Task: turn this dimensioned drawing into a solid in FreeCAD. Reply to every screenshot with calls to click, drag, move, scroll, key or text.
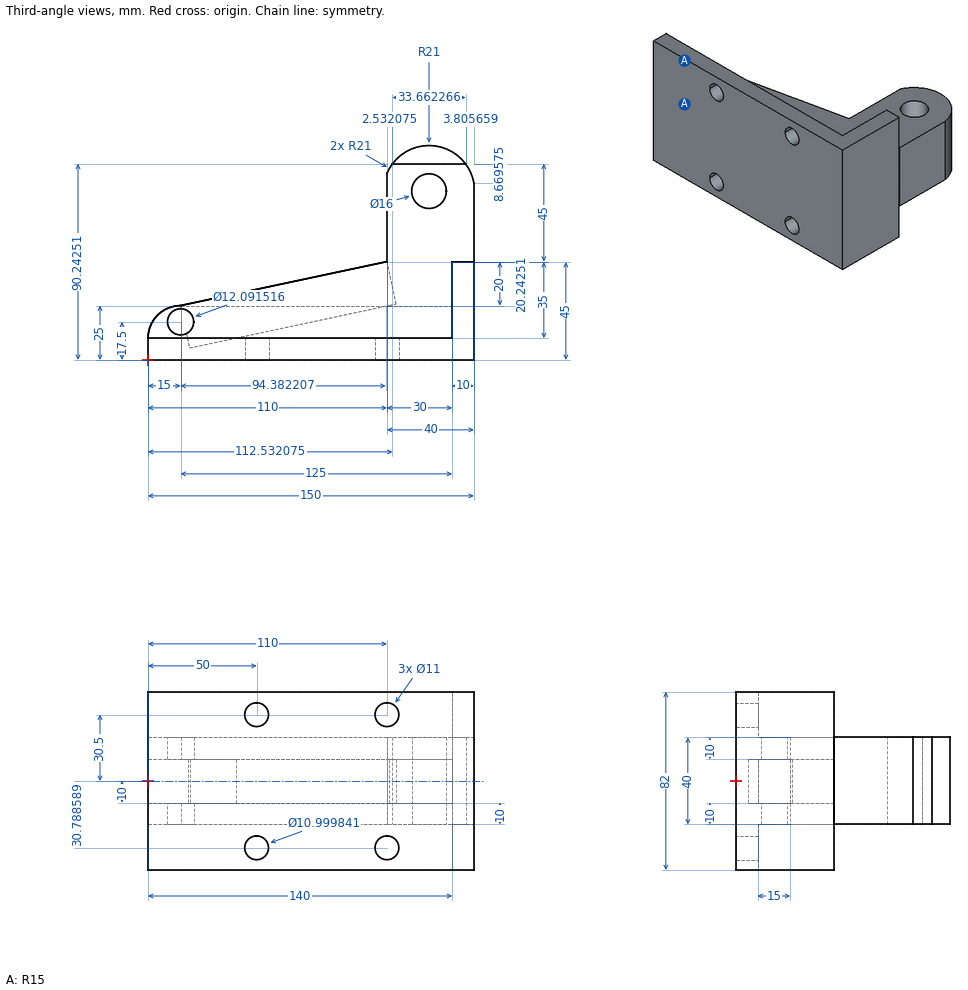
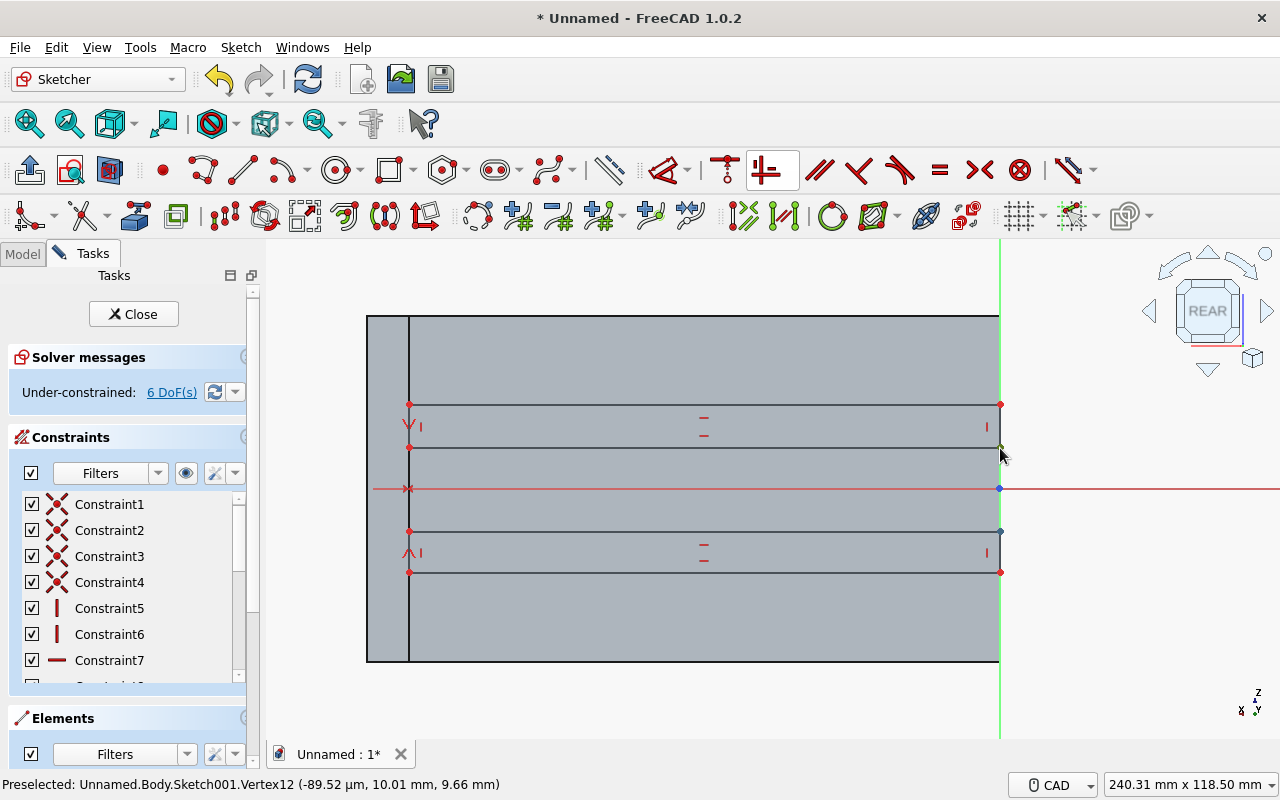
click(470, 489)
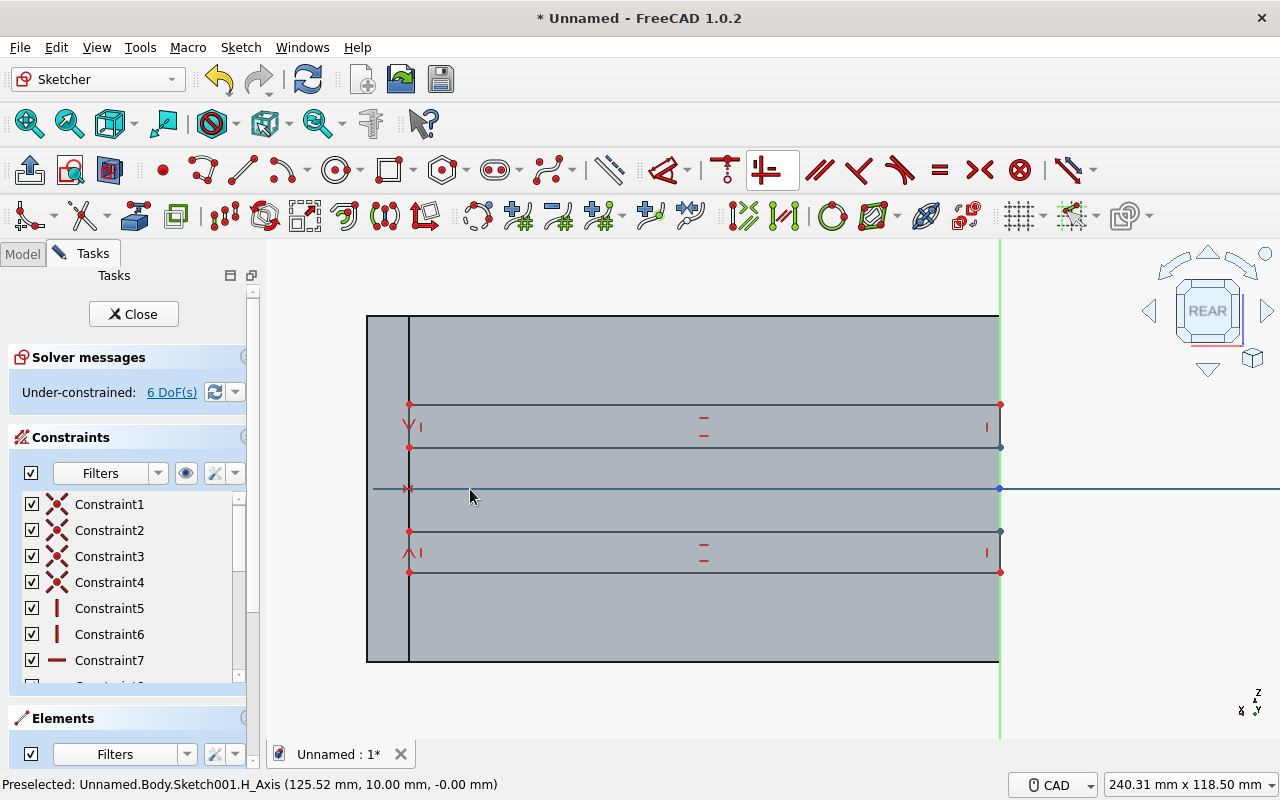
key(s)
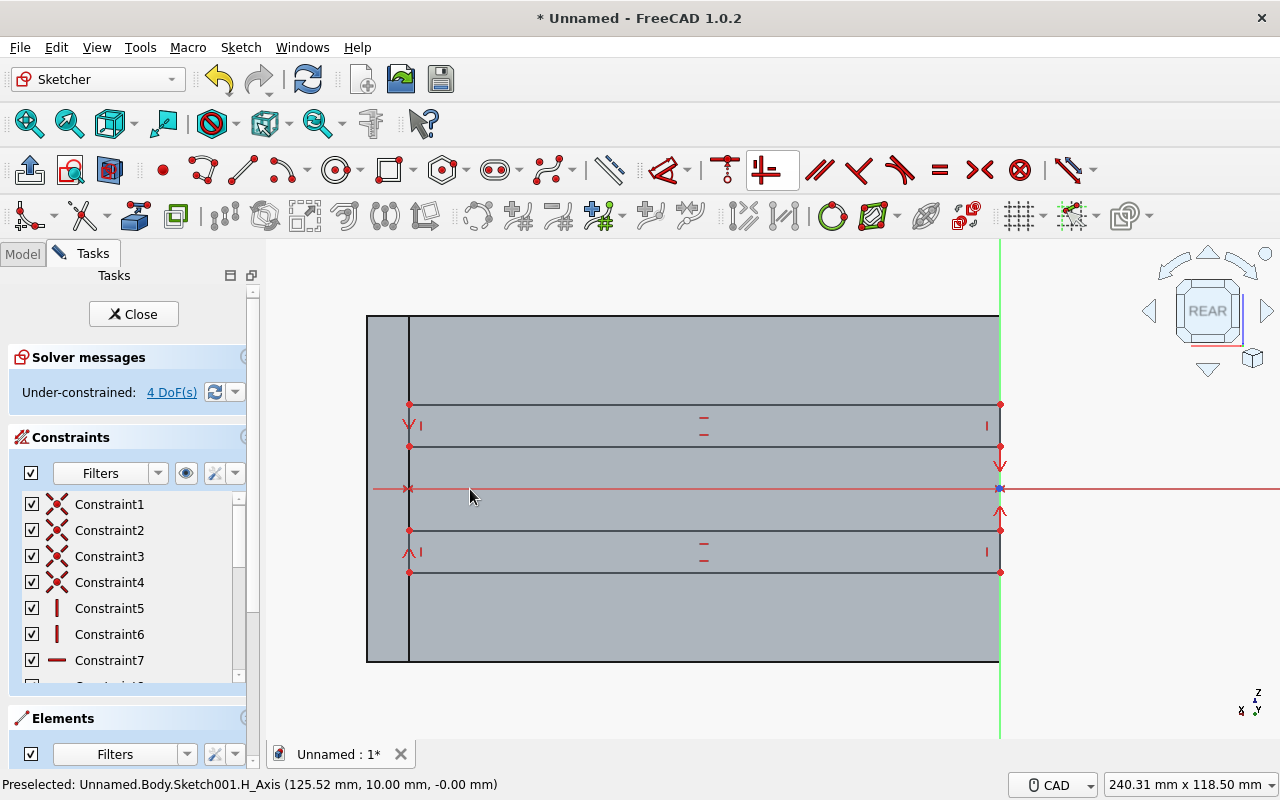
click(1000, 573)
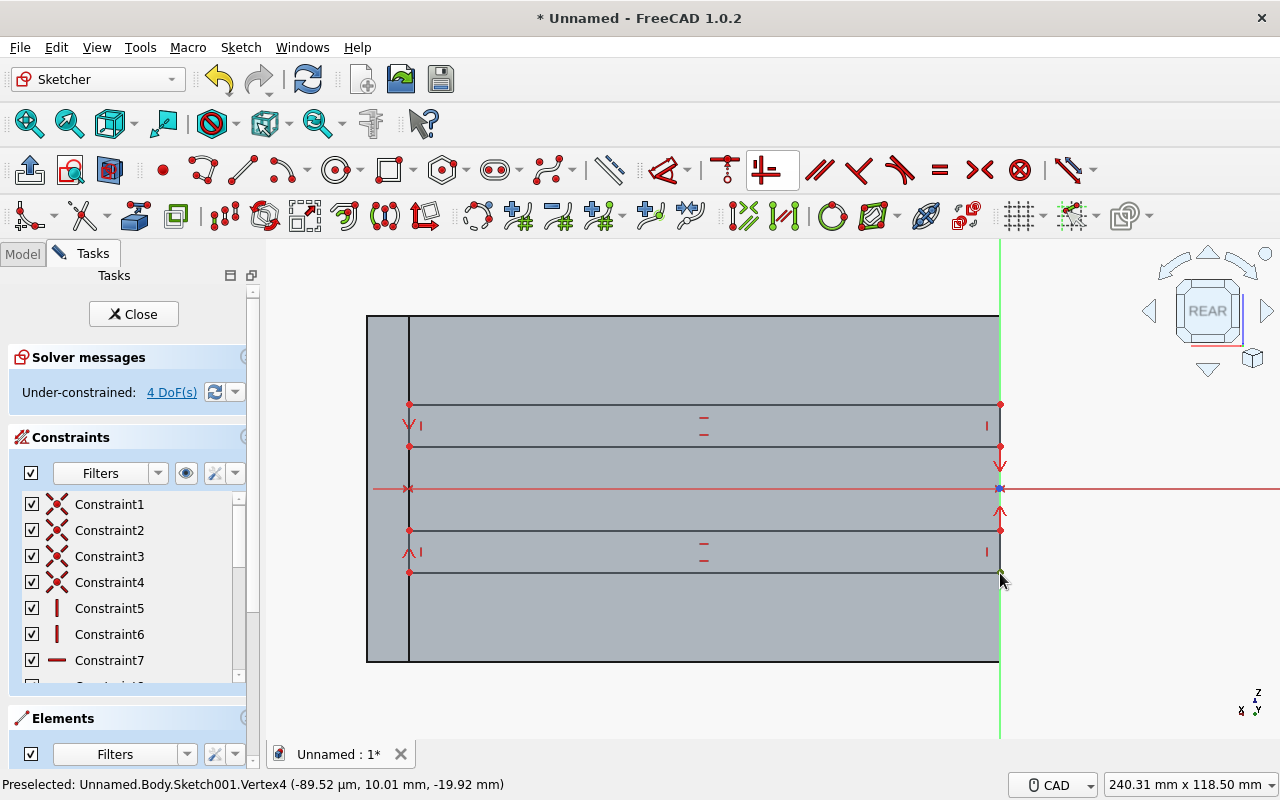
click(1000, 679)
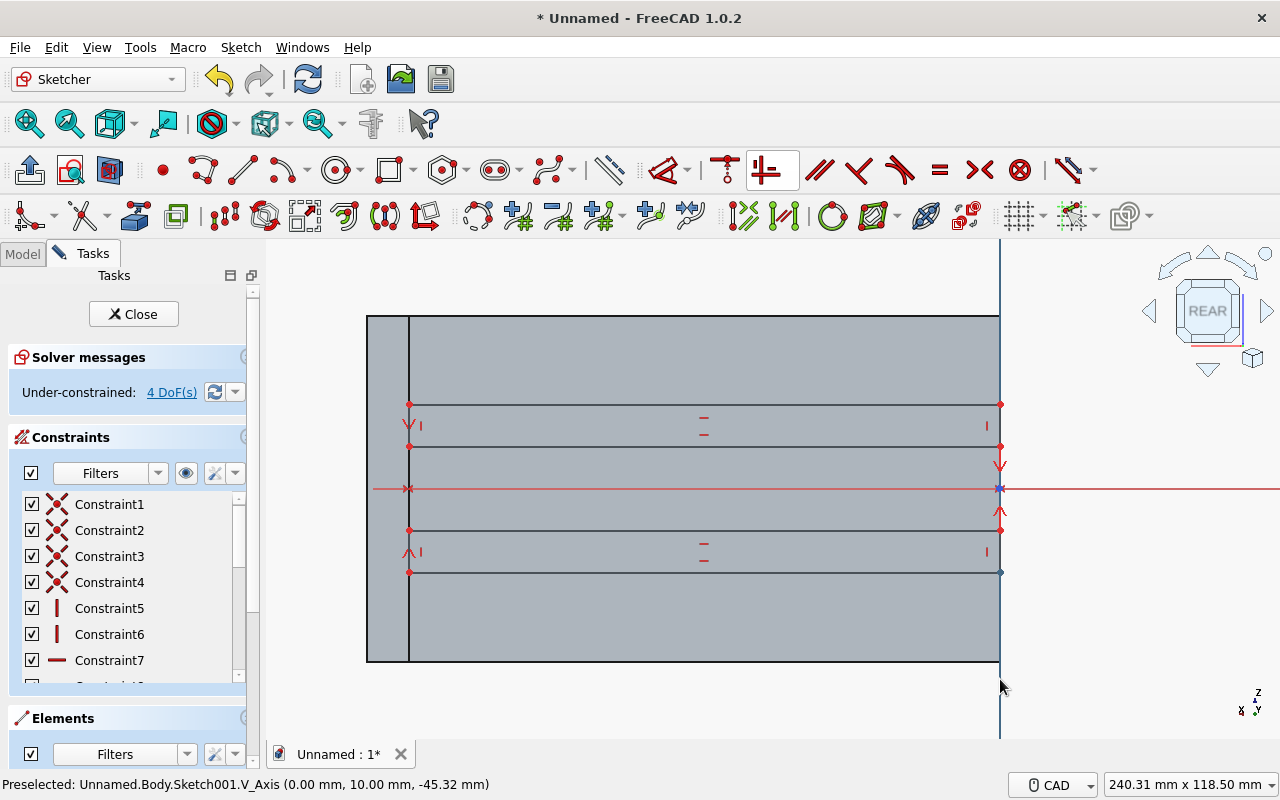
click(726, 170)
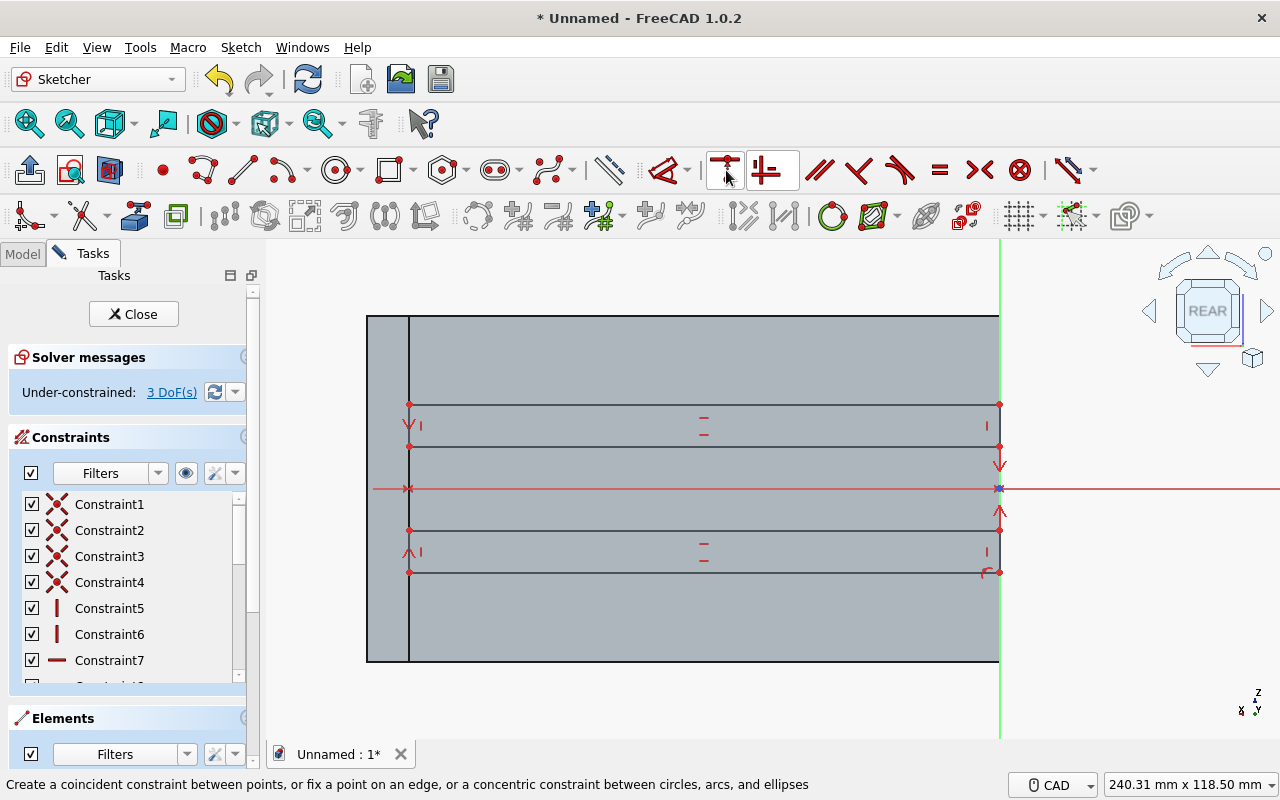
key(d)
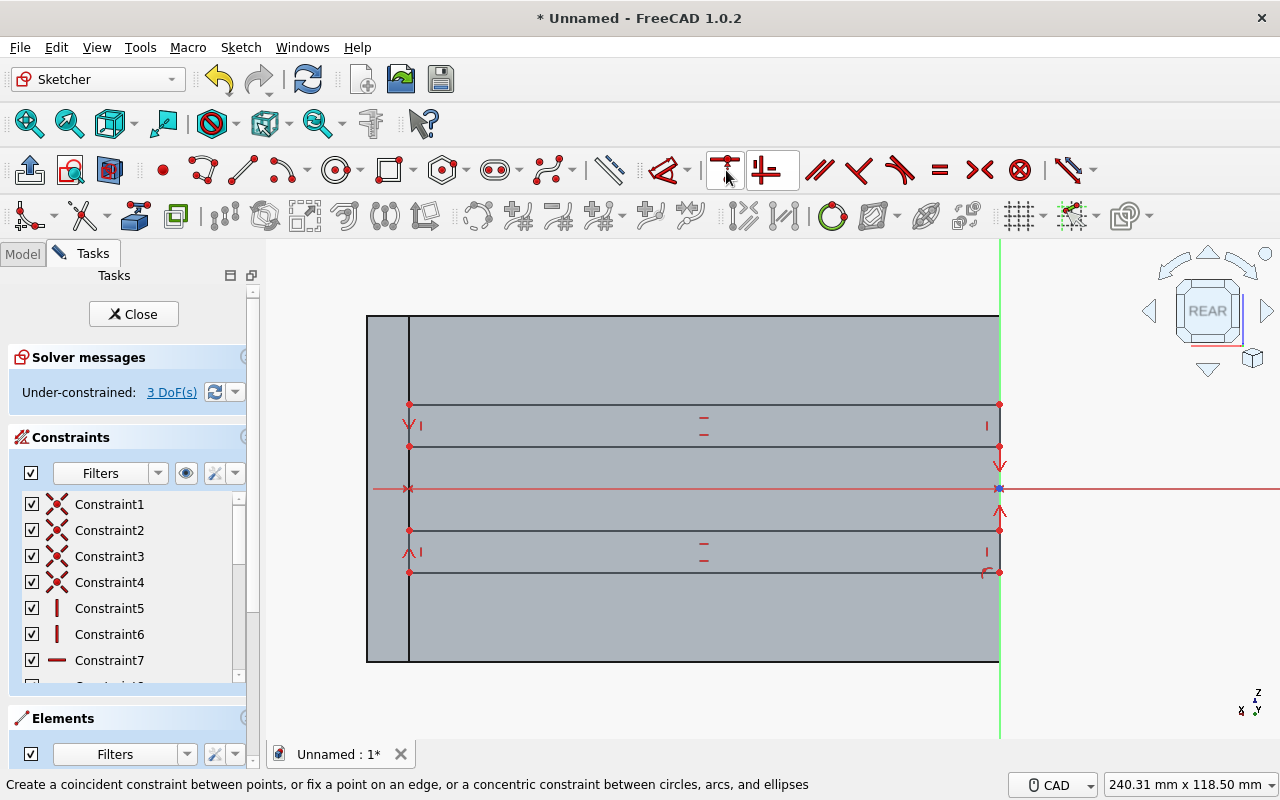
click(409, 543)
click(375, 552)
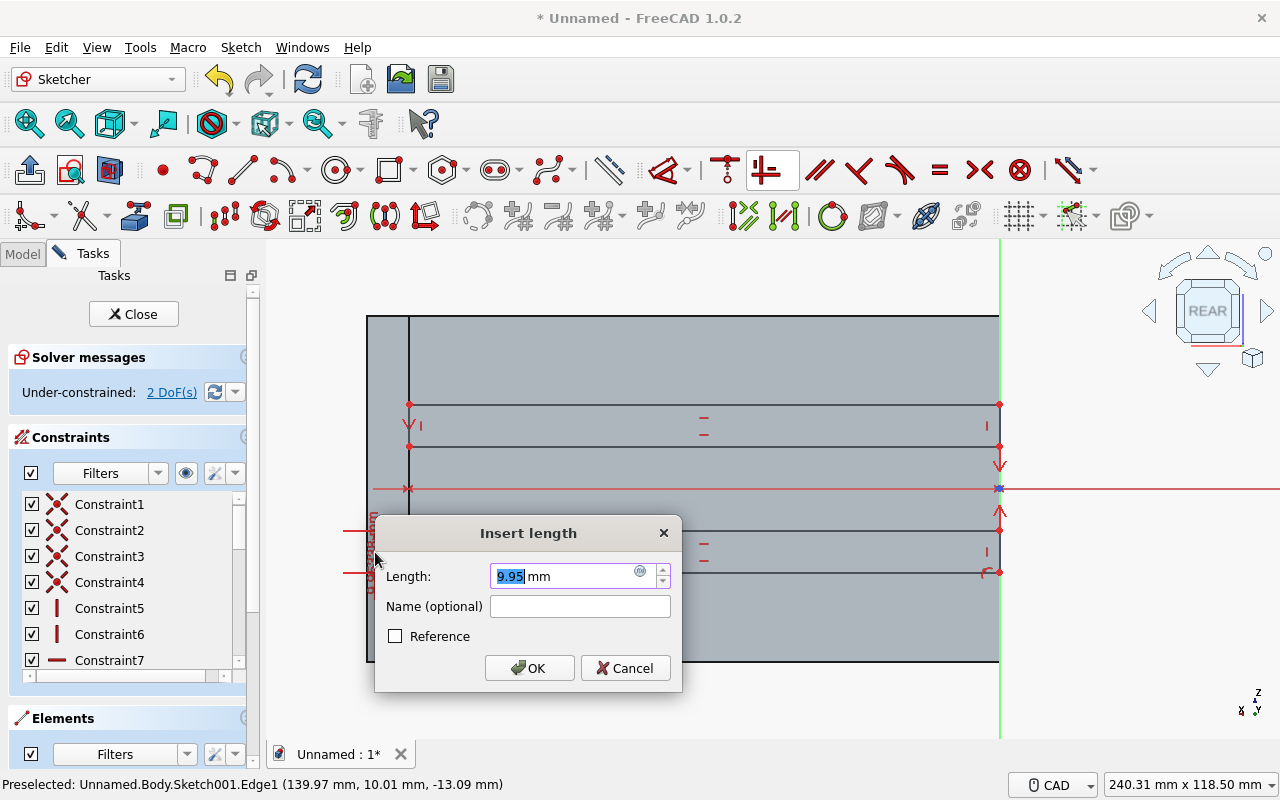
text(10)
key(Return)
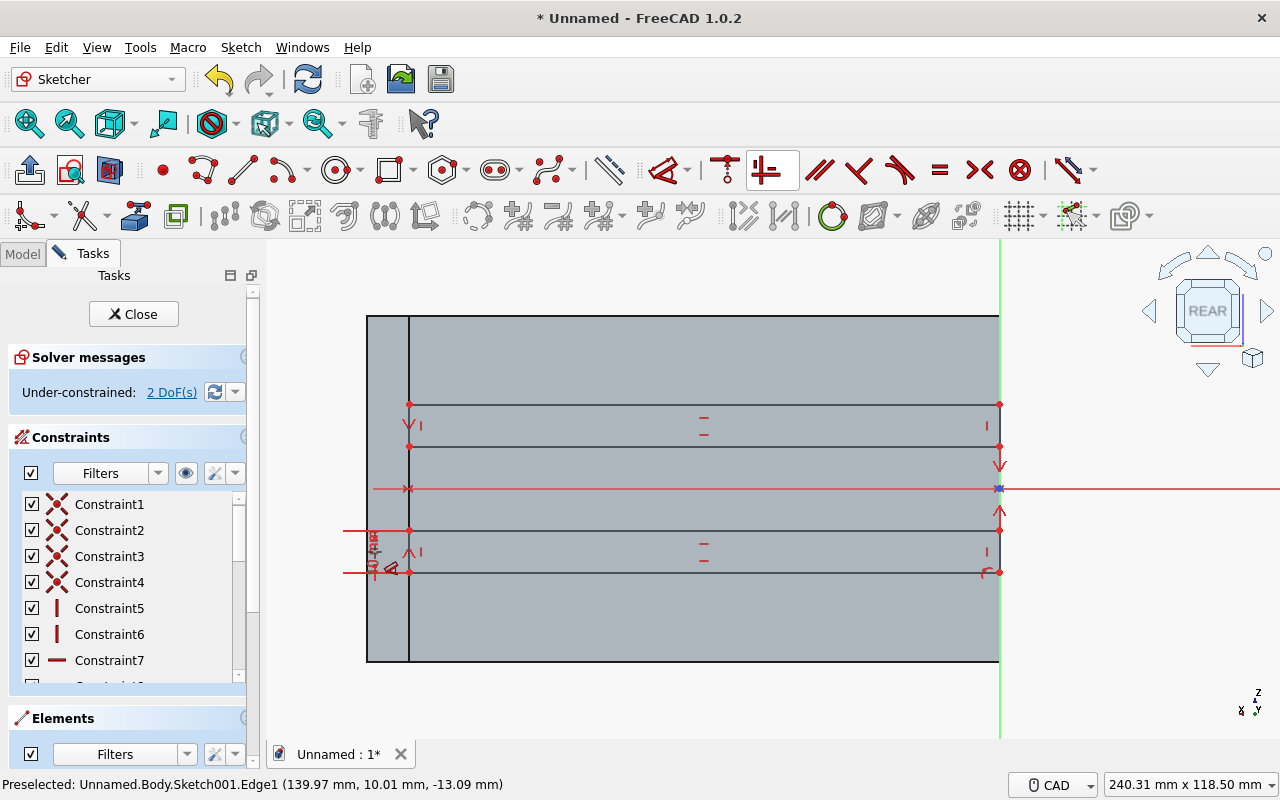
click(586, 573)
click(704, 607)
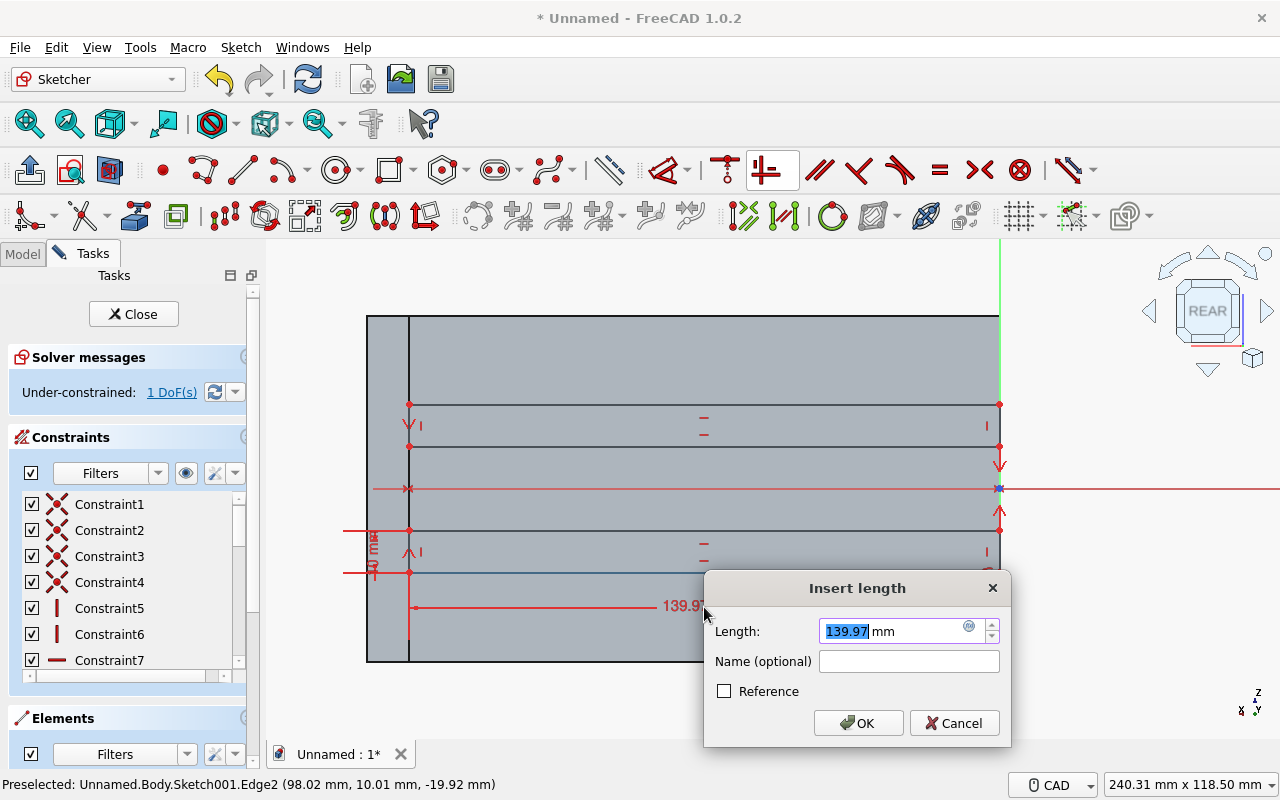
text(140)
key(Return)